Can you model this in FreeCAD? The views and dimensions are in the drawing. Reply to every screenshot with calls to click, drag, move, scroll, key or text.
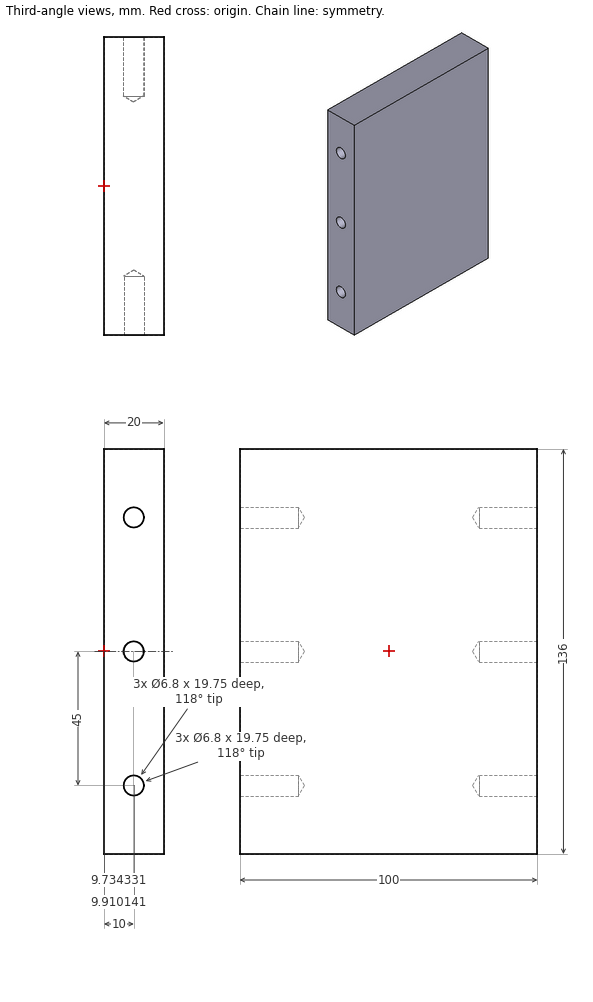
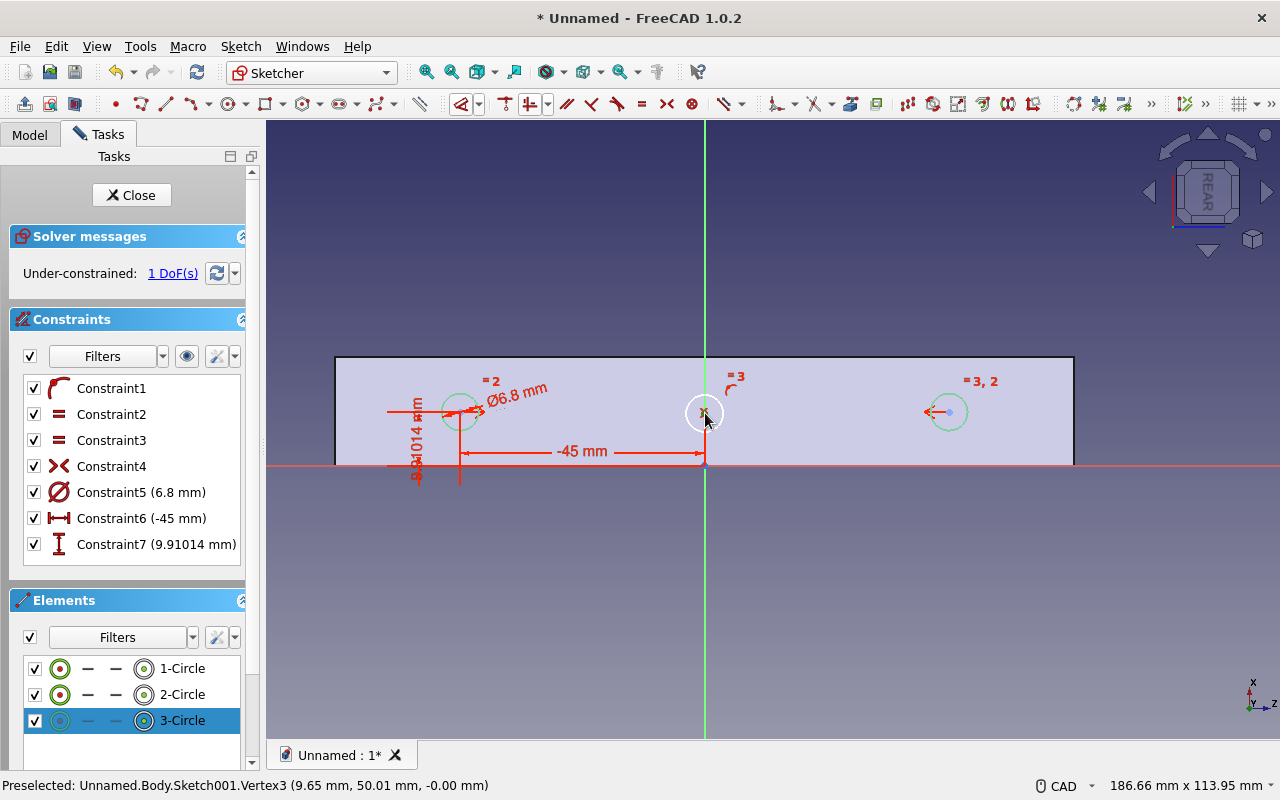
click(478, 104)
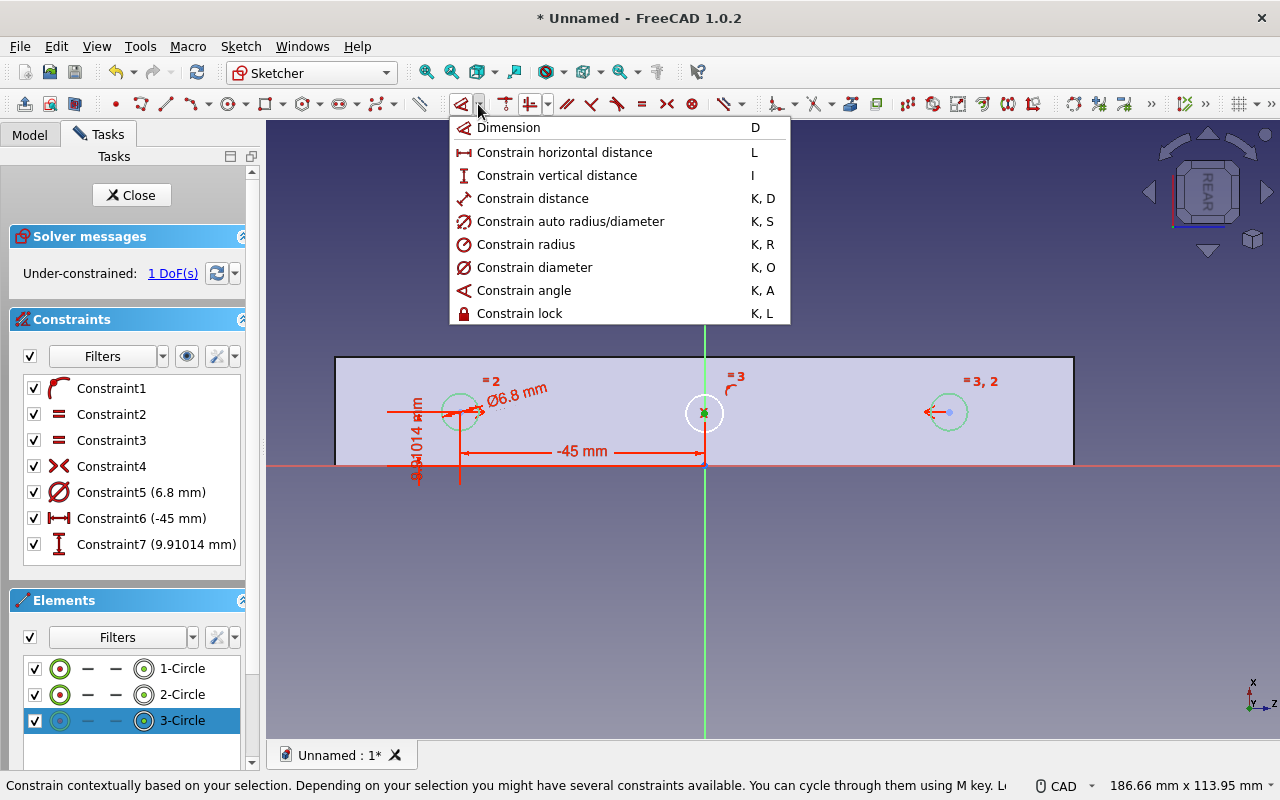
click(620, 176)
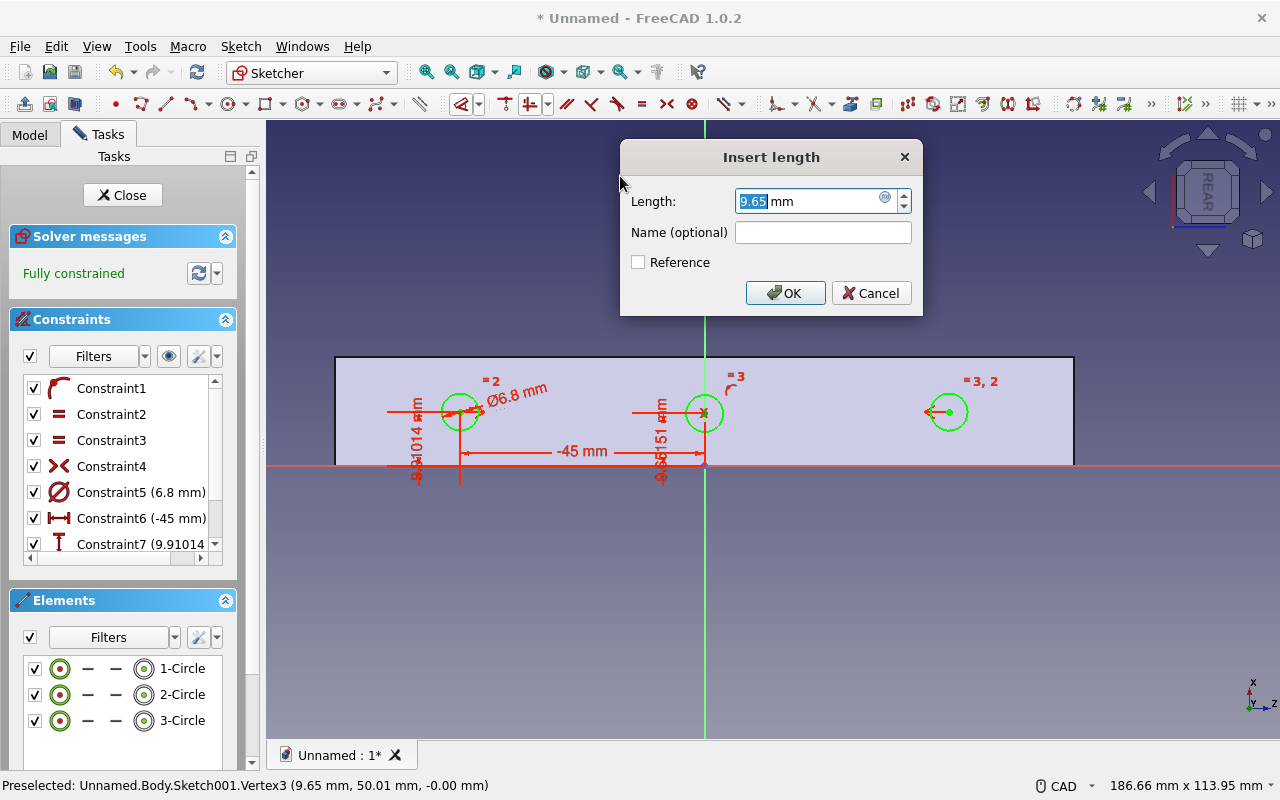
text(9.734331)
key(Return)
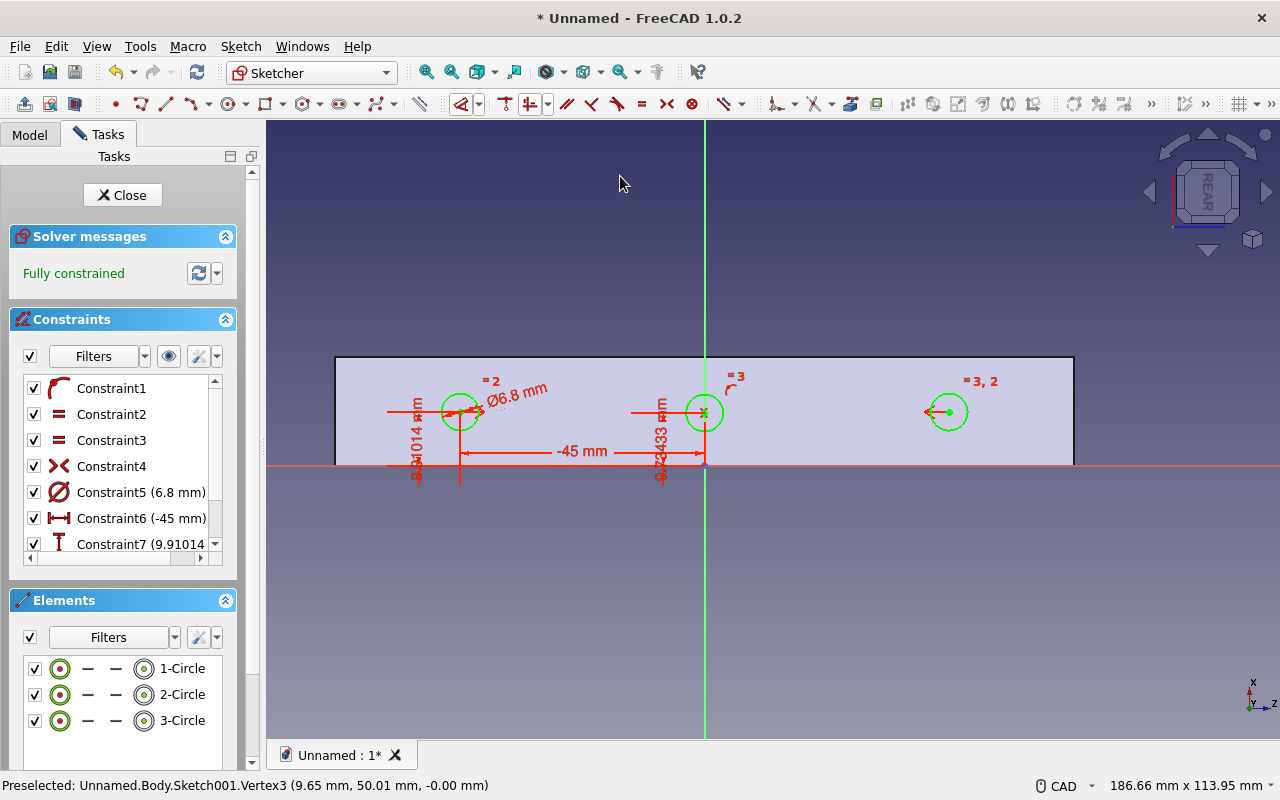
click(123, 195)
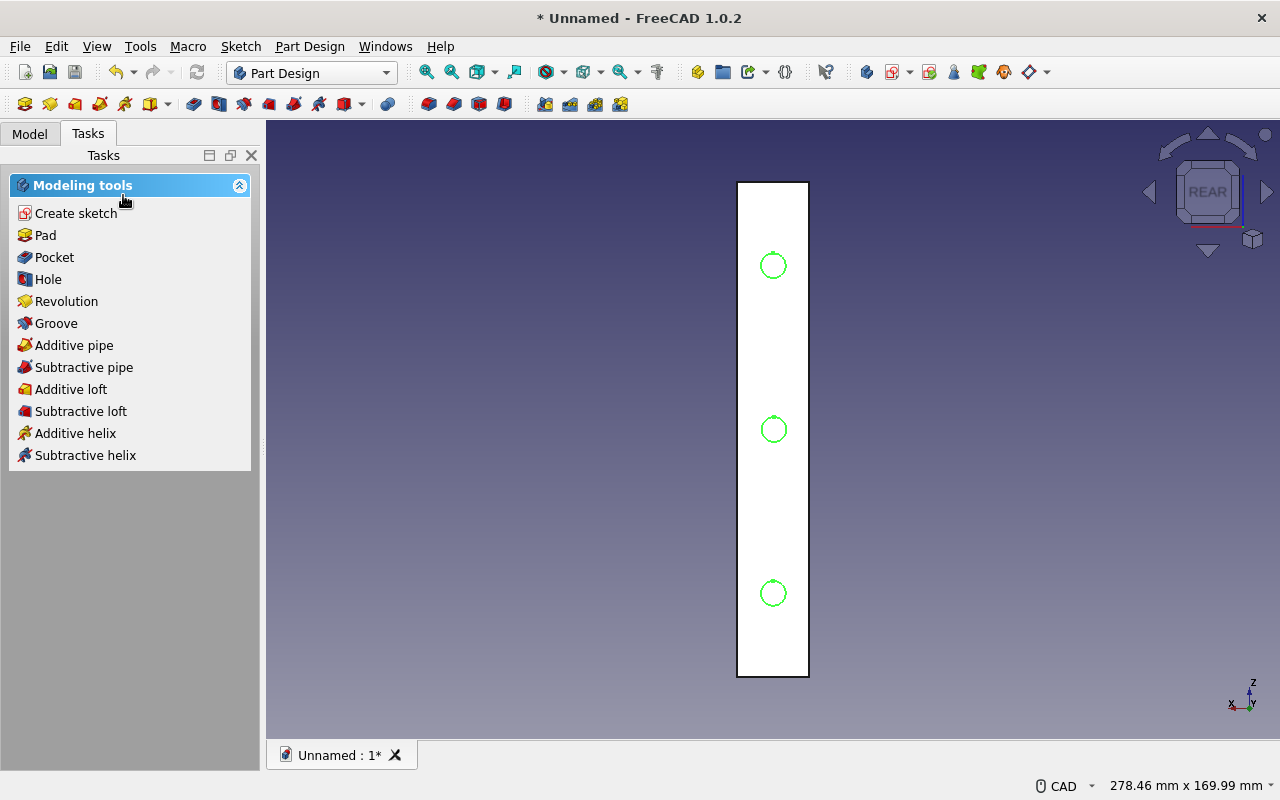
click(219, 104)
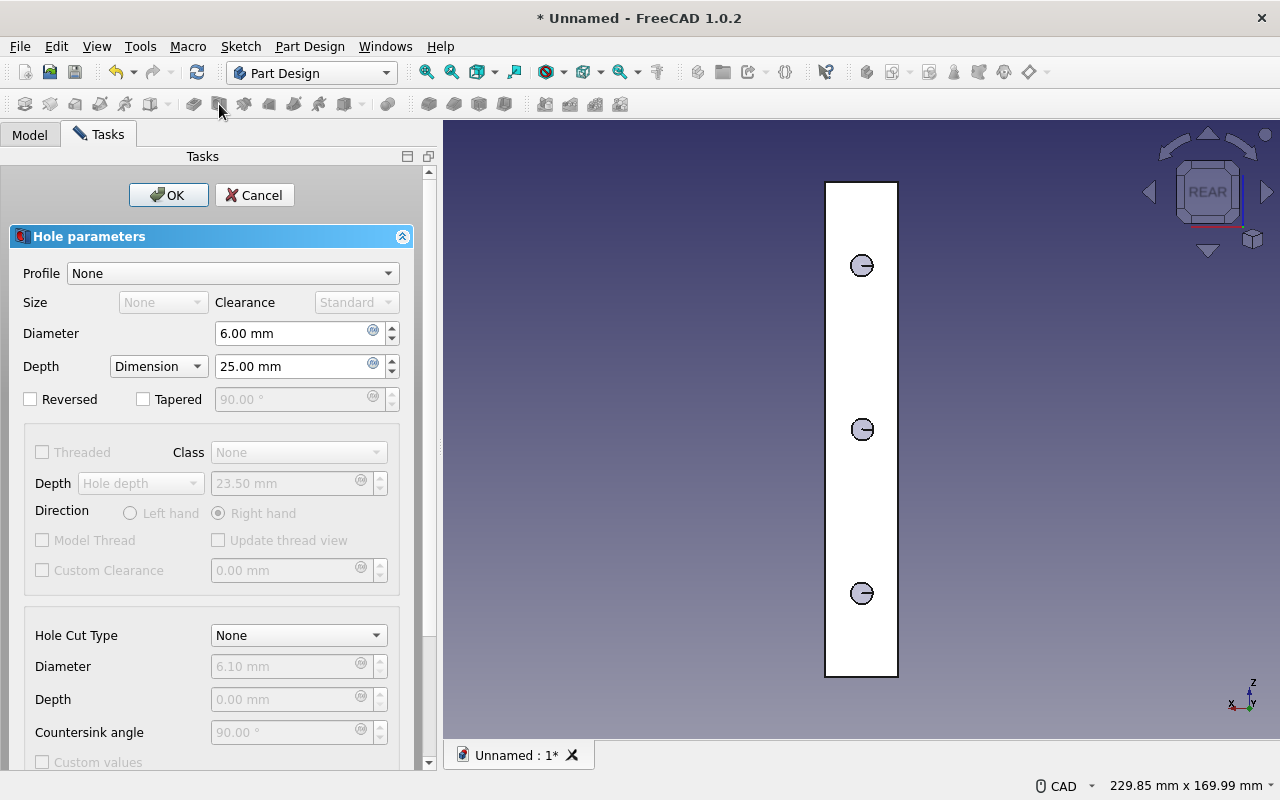
triple_click(300, 334)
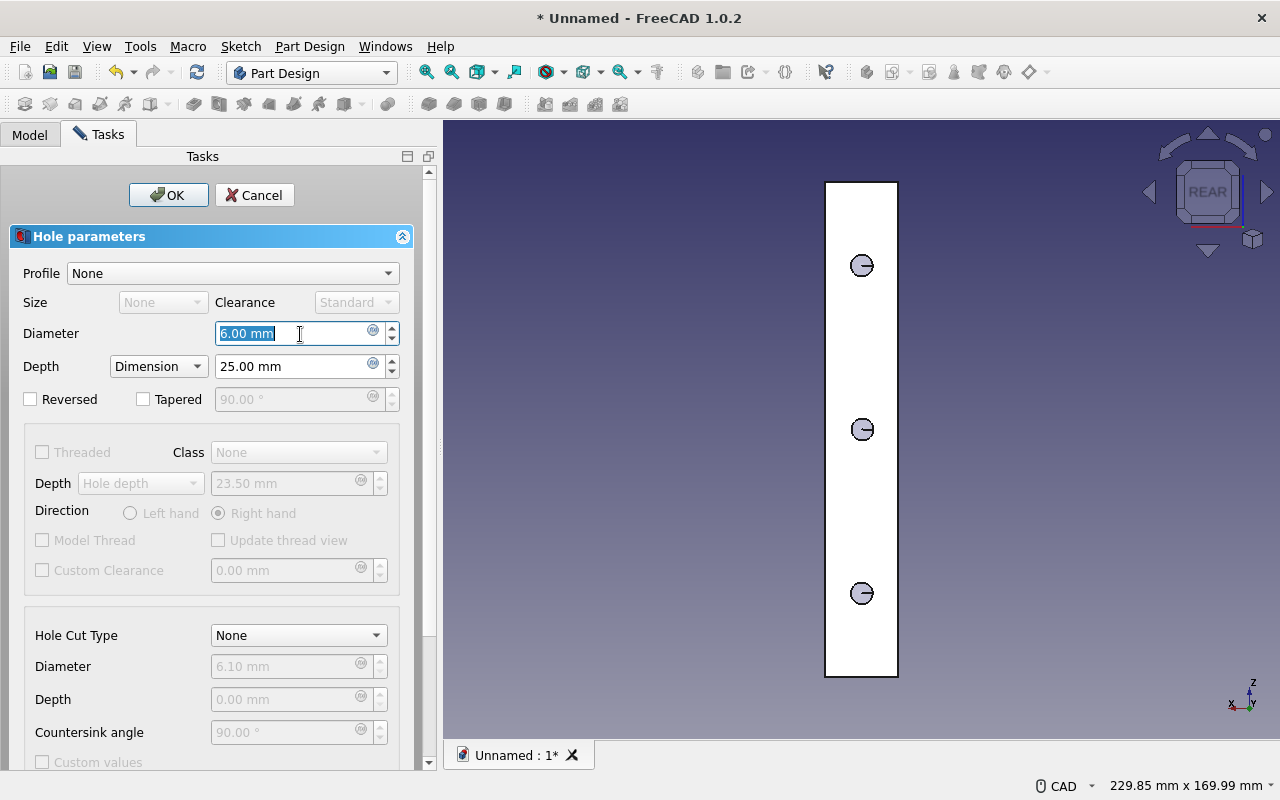
text(6.8)
key(Tab)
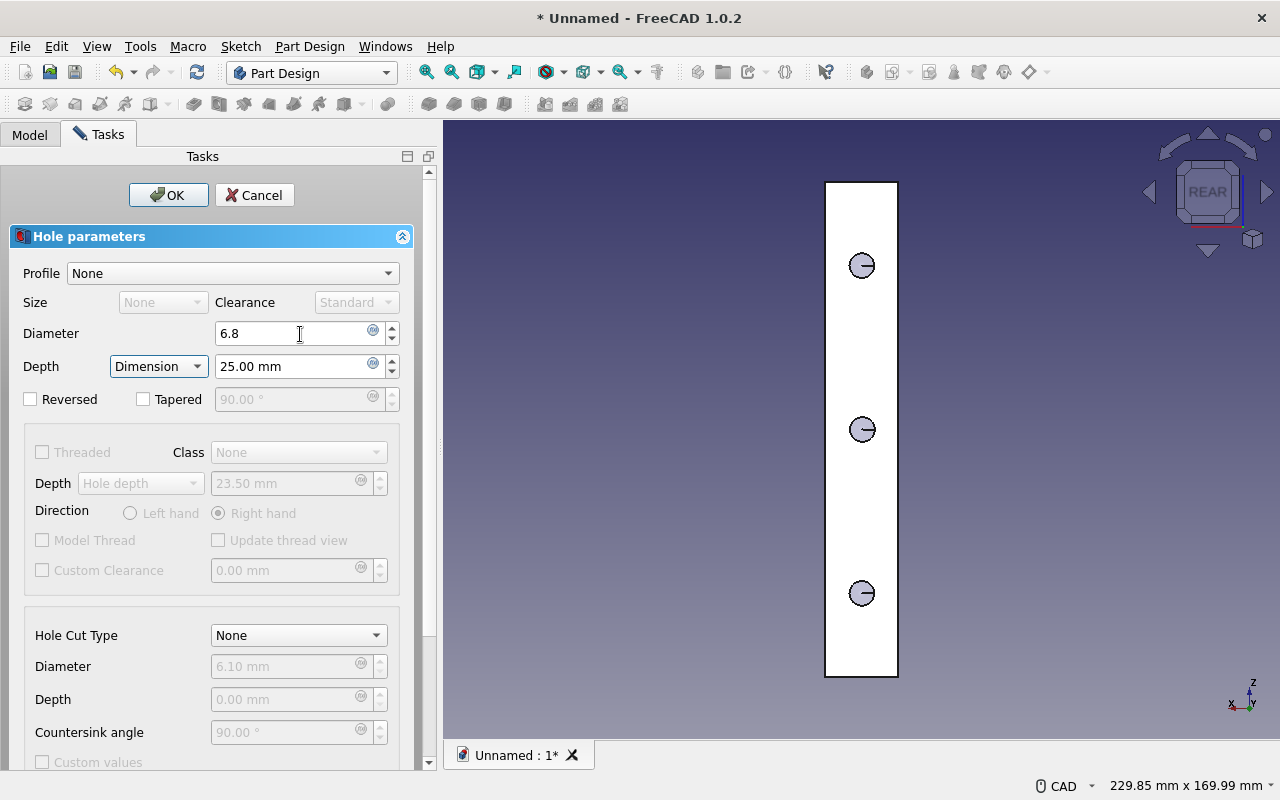
triple_click(300, 366)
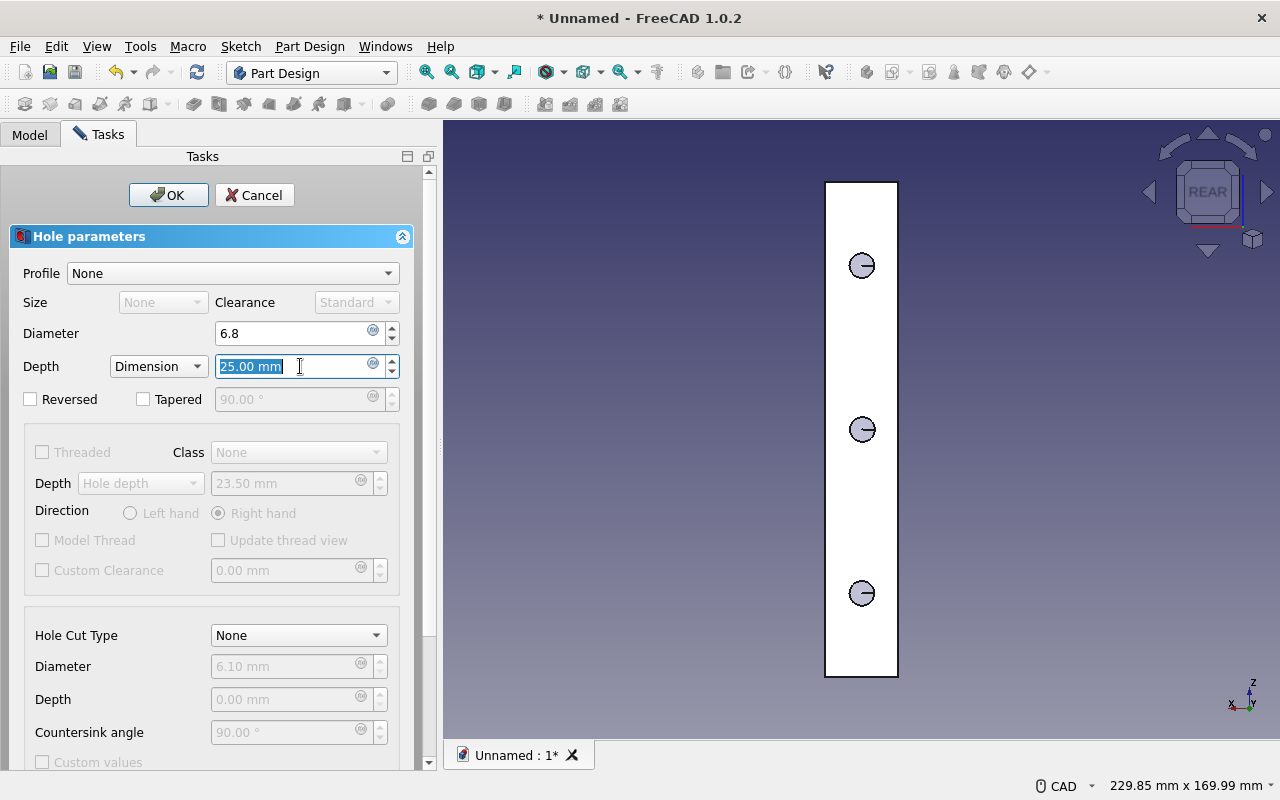
text(19.75)
key(Tab)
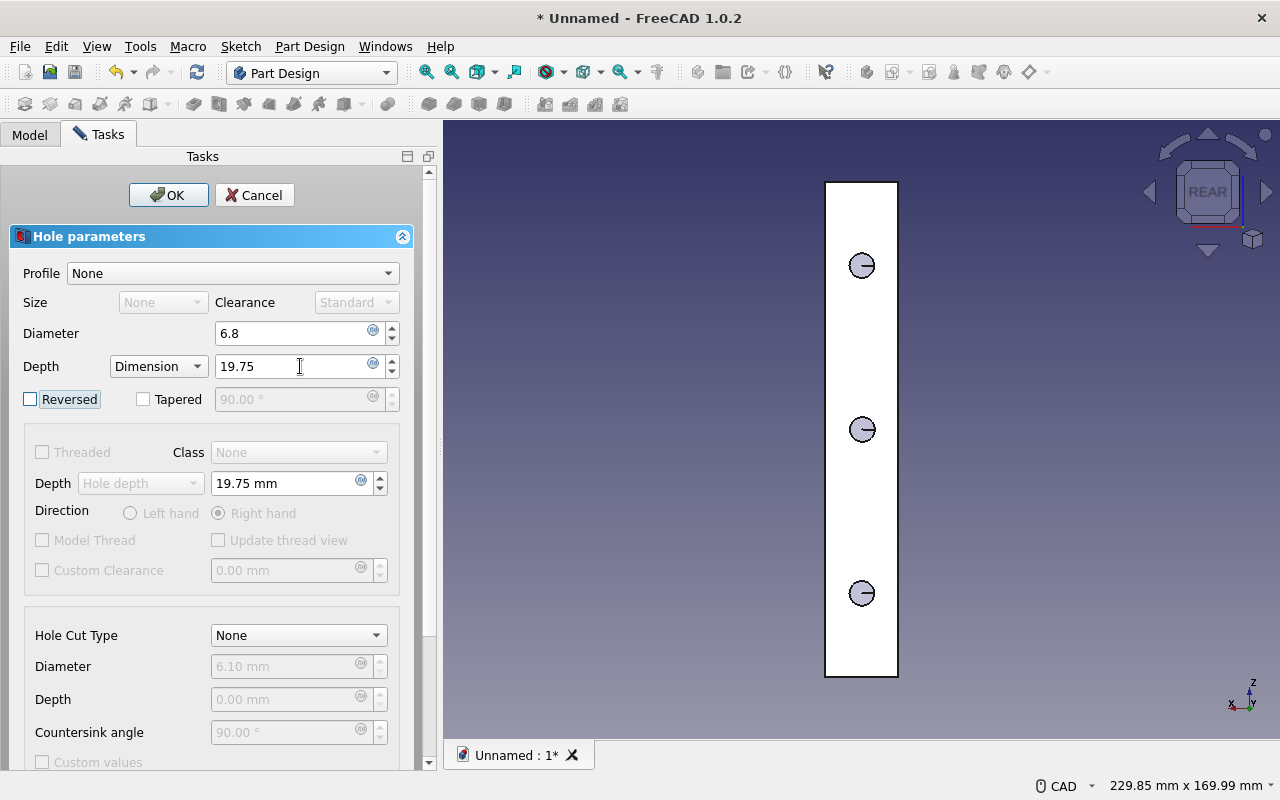
click(169, 195)